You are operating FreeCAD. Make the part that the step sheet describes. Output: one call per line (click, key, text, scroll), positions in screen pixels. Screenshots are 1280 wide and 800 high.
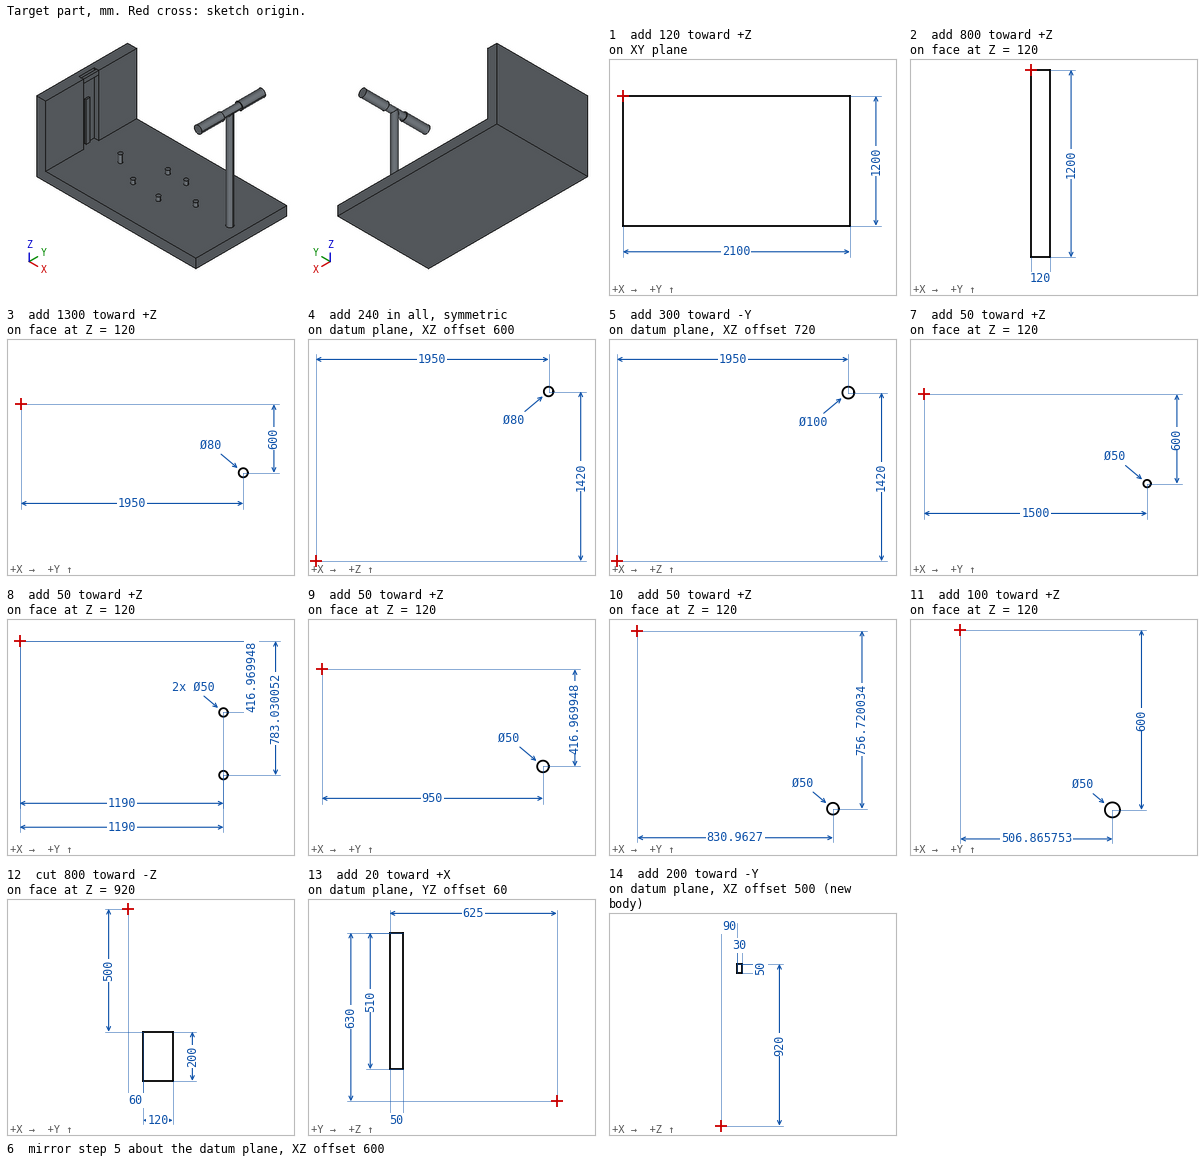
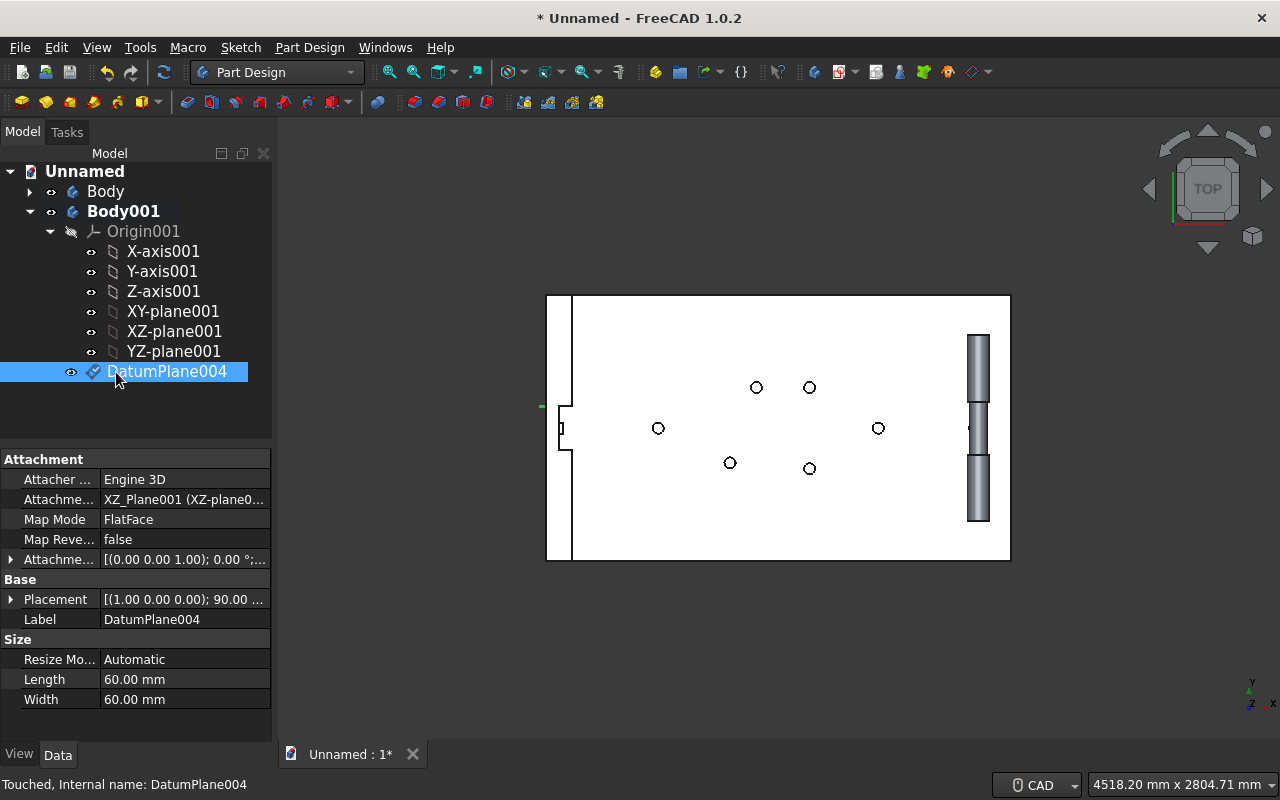
click(840, 72)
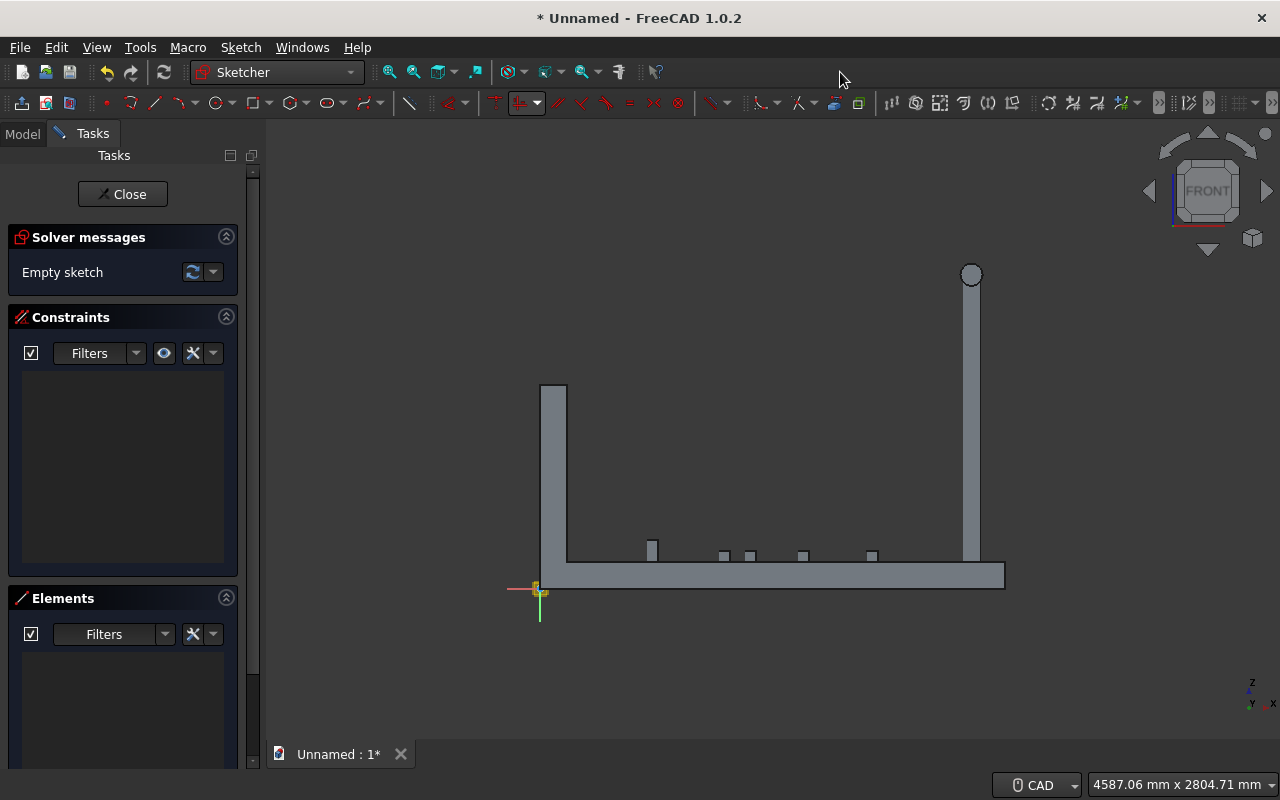
scroll(556, 389, up, 15)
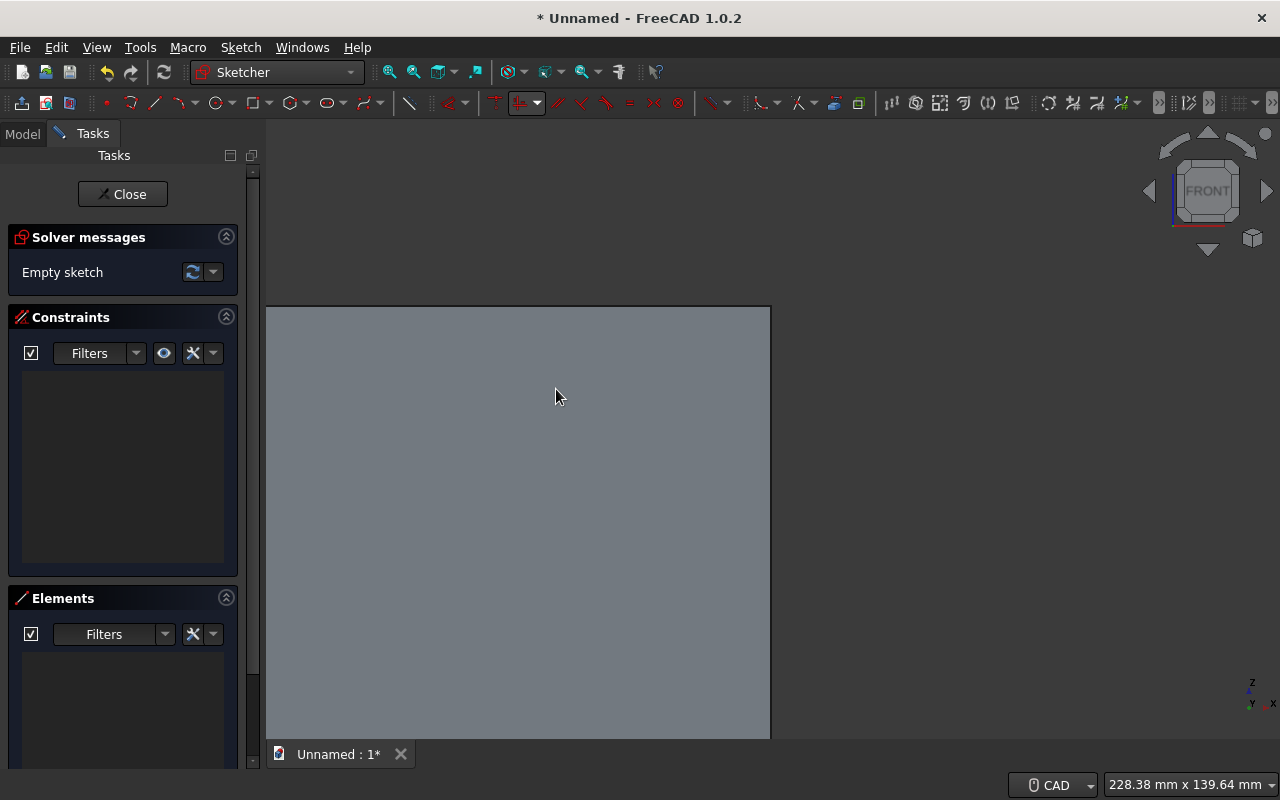
scroll(705, 403, up, 3)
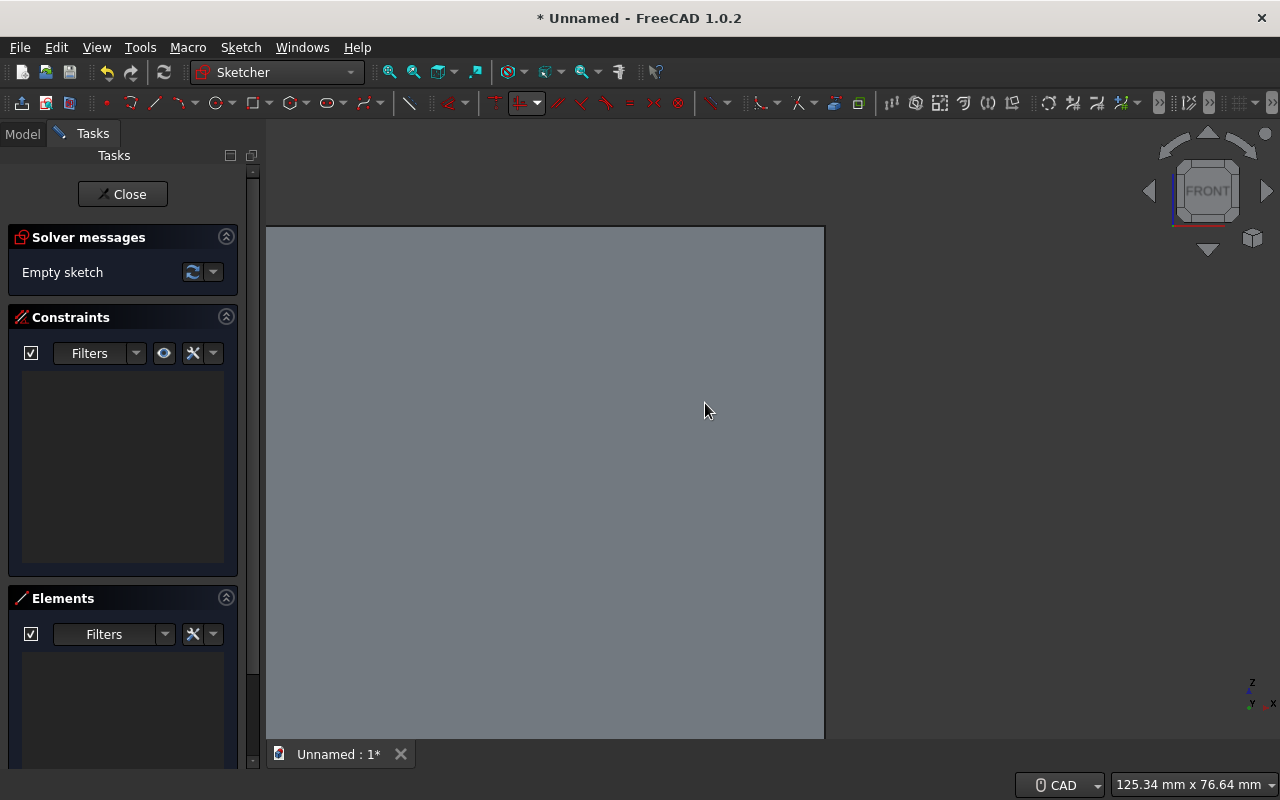
click(254, 104)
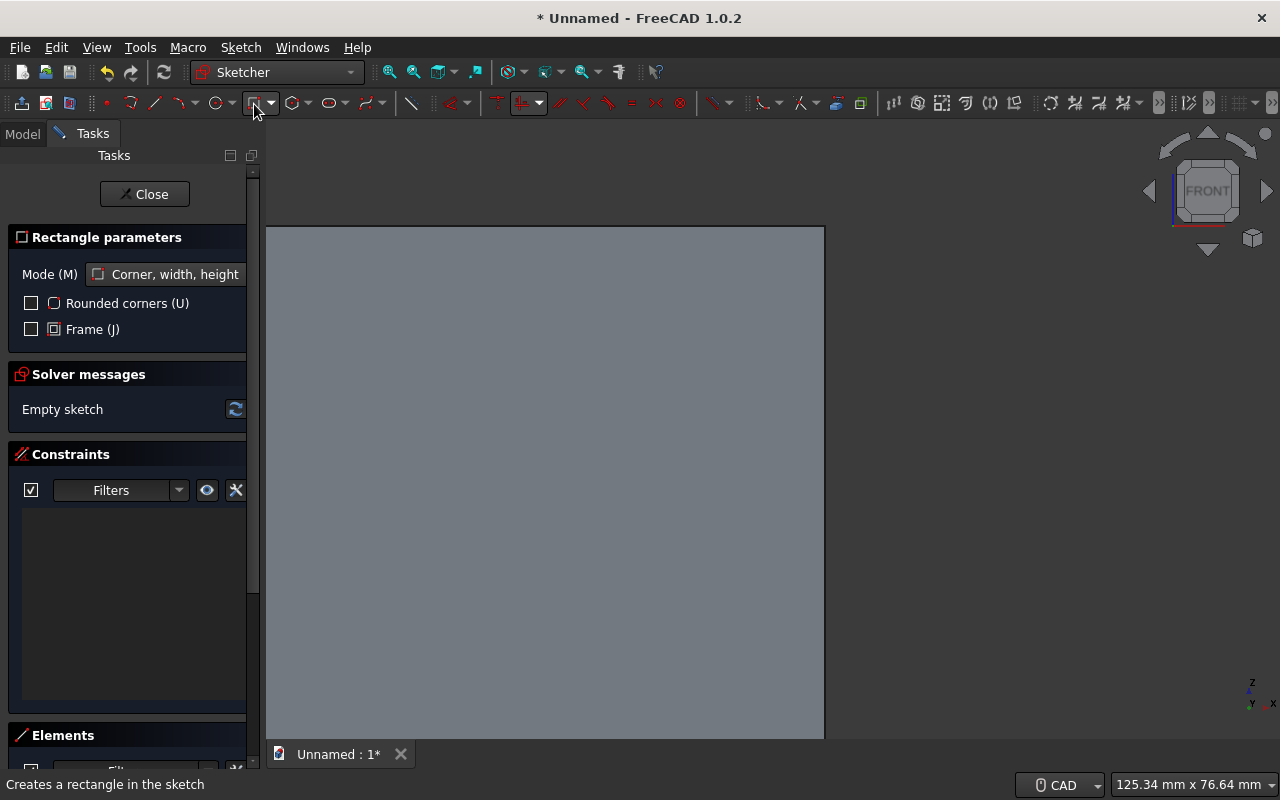
click(583, 226)
move(825, 631)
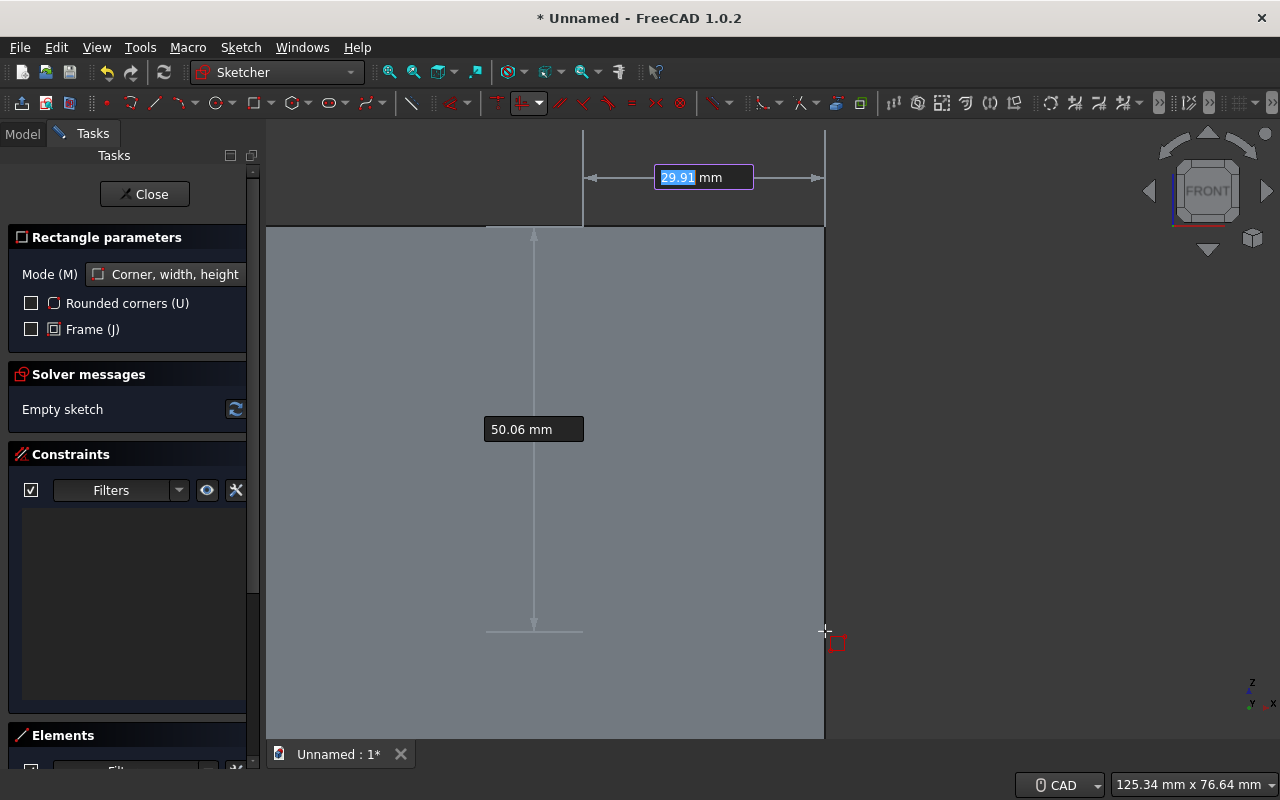
text(30)
key(Tab)
text(50)
key(Return)
key(Escape)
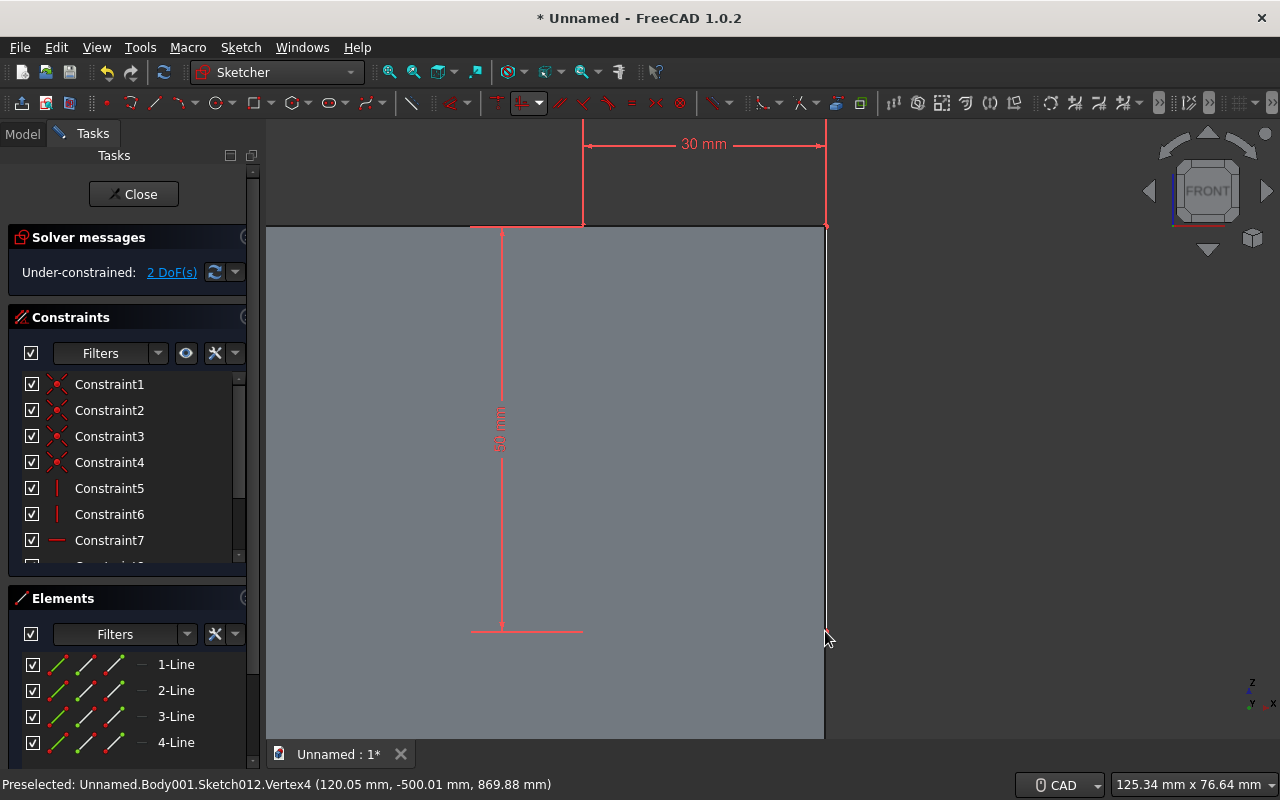
click(450, 104)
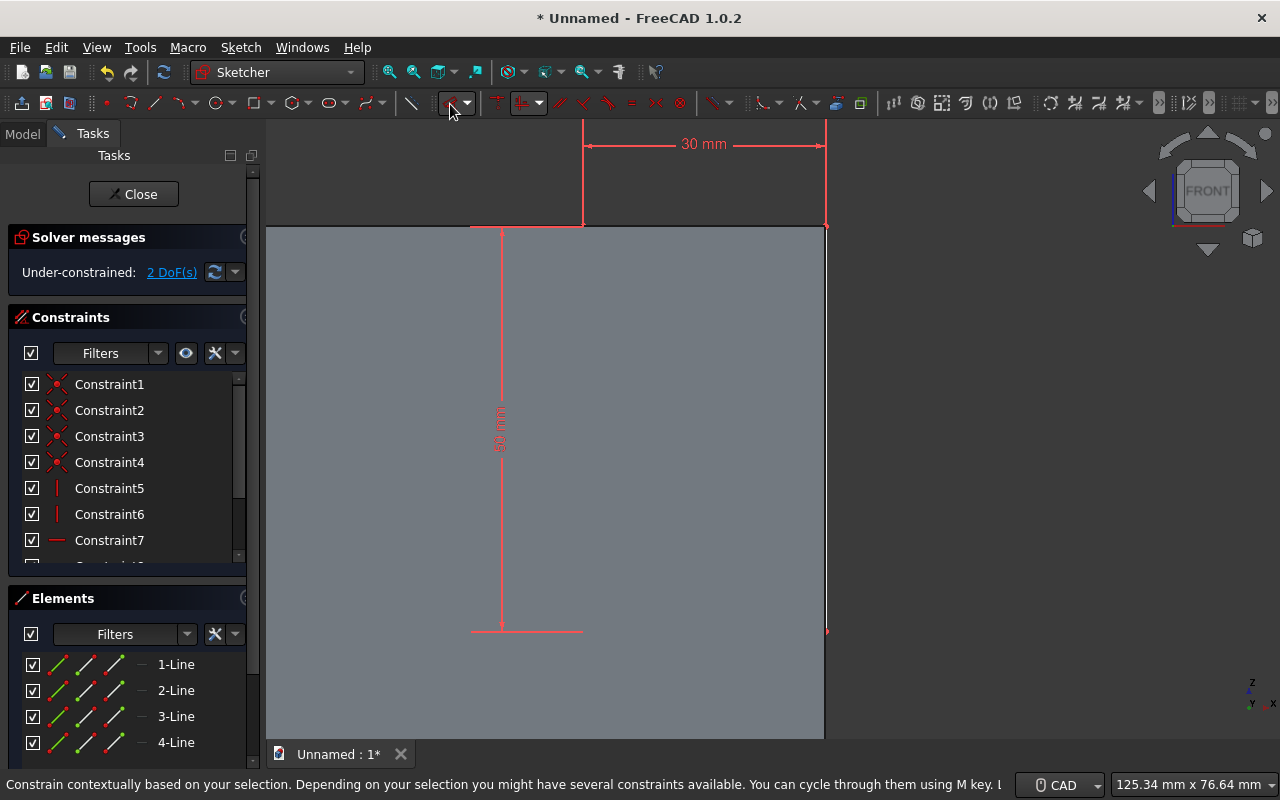
click(583, 227)
click(439, 193)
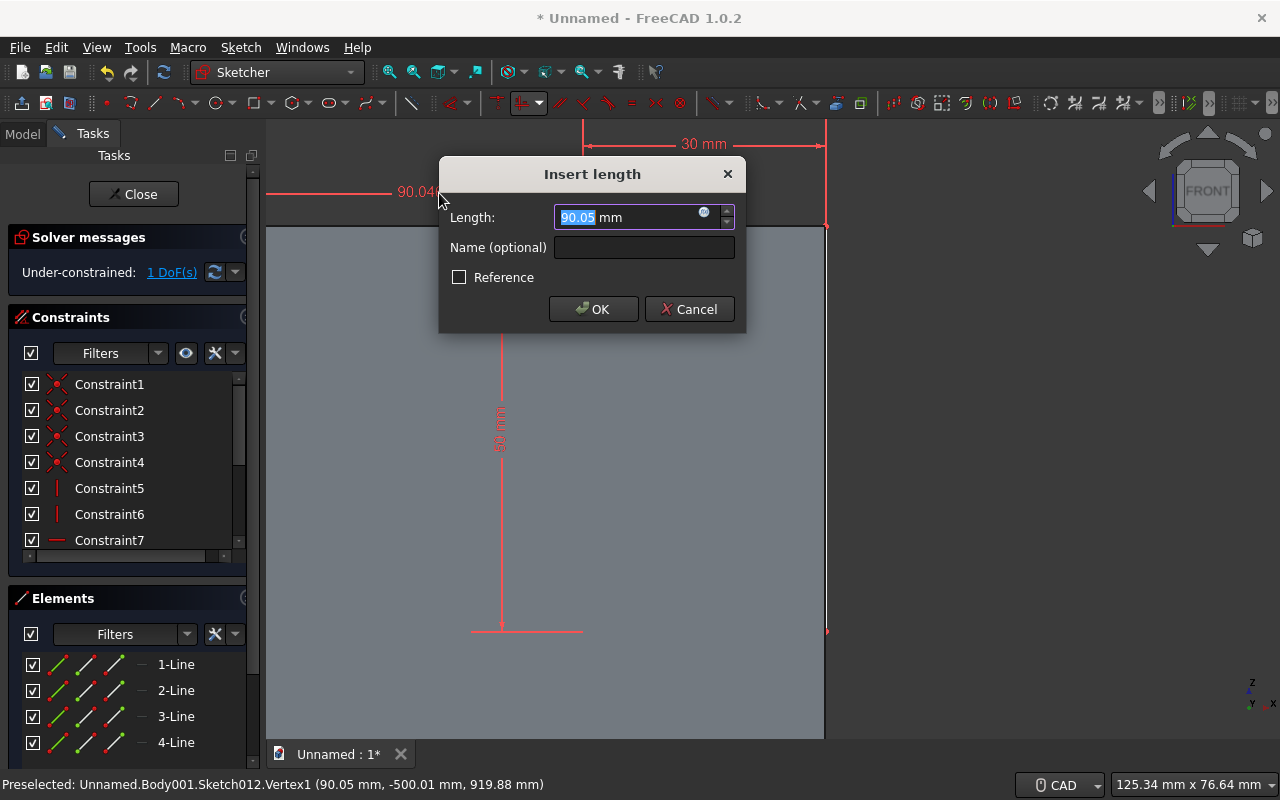
text(90)
key(Return)